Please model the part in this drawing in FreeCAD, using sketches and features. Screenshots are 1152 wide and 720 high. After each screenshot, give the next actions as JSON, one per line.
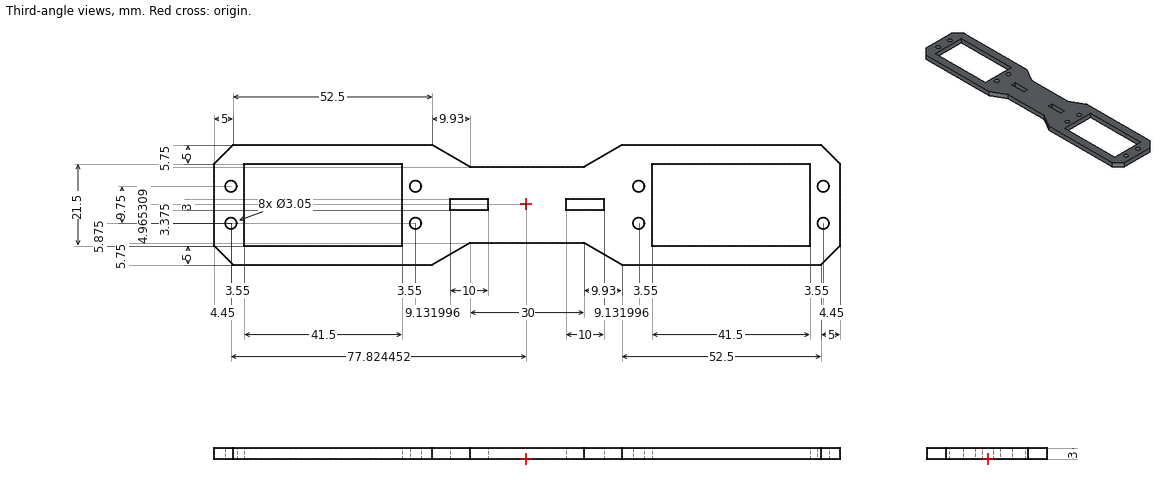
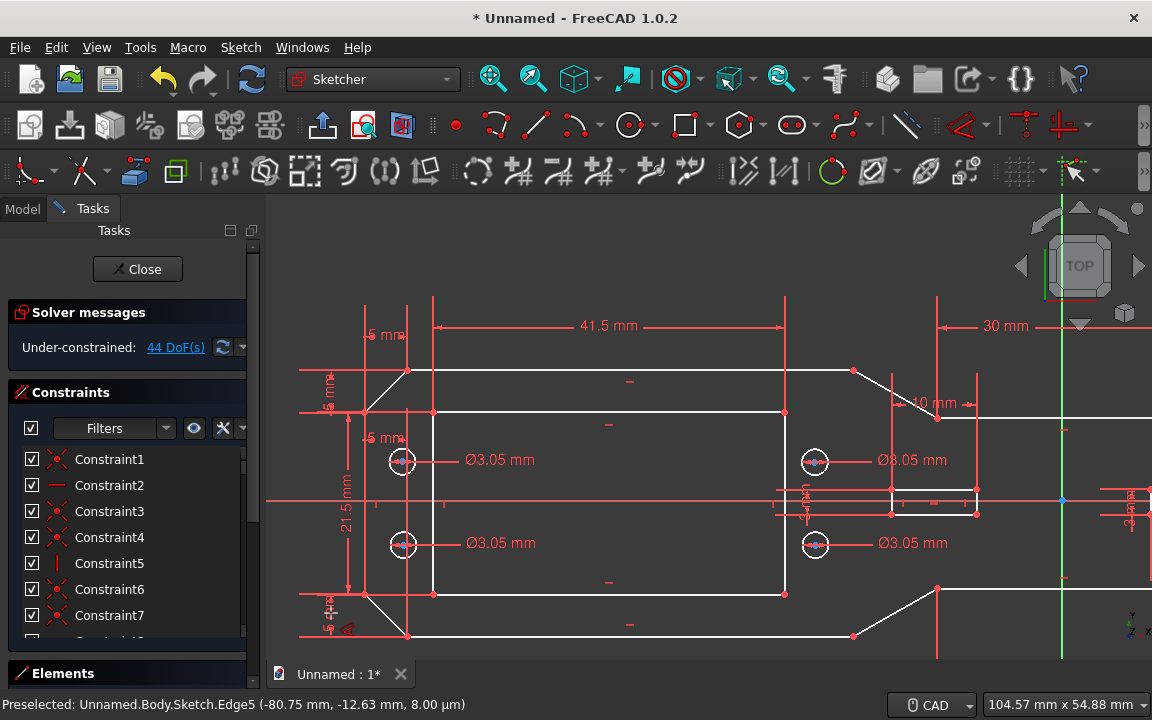
{"action": "scroll", "coordinate": [394, 383], "scroll_direction": "down", "scroll_amount": 5}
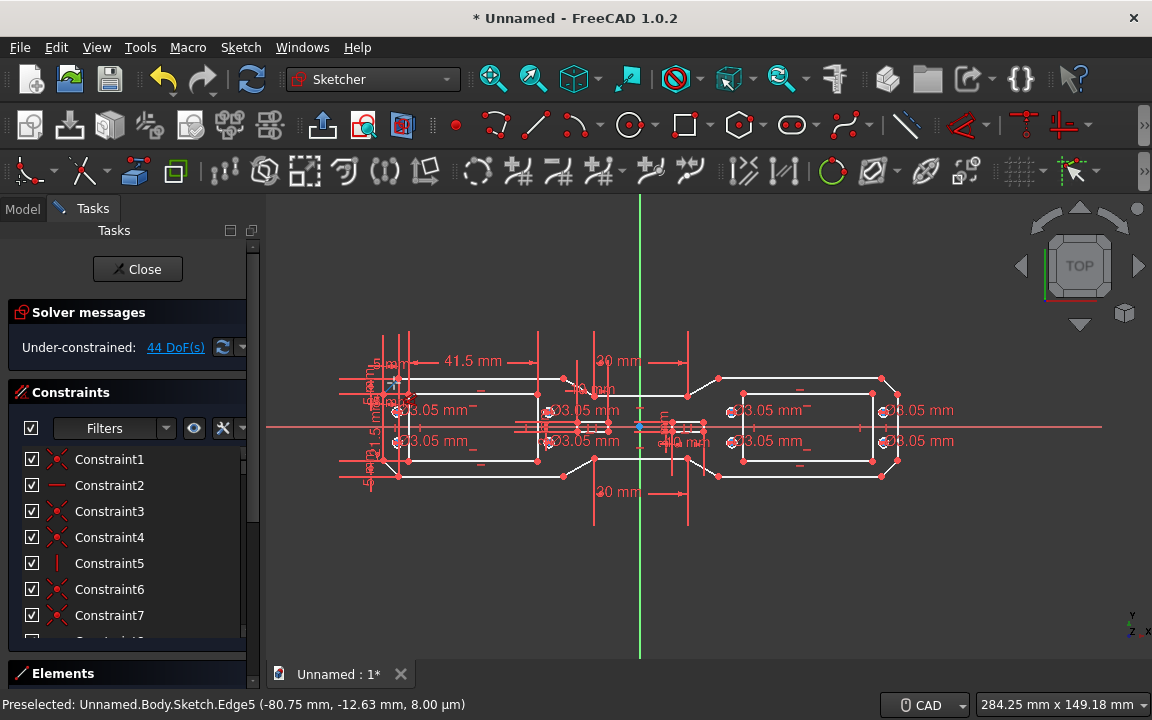
{"action": "scroll", "coordinate": [887, 472], "scroll_direction": "up", "scroll_amount": 5}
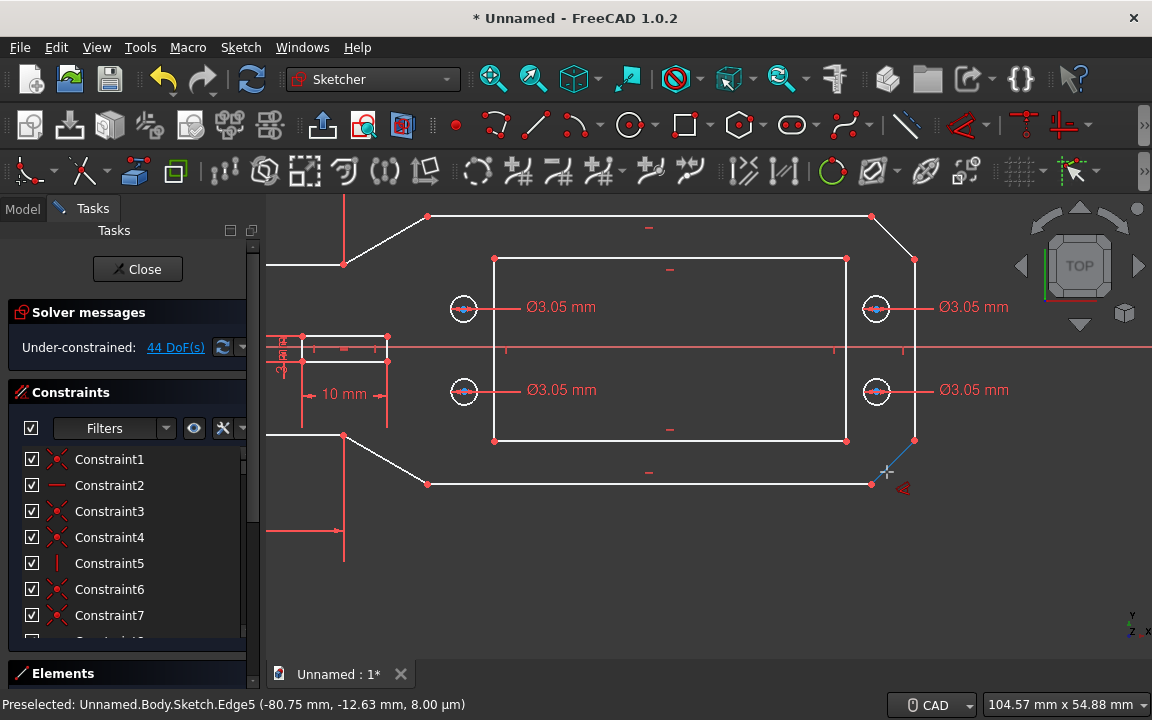
{"action": "left_click", "coordinate": [885, 471]}
{"action": "left_click", "coordinate": [893, 518]}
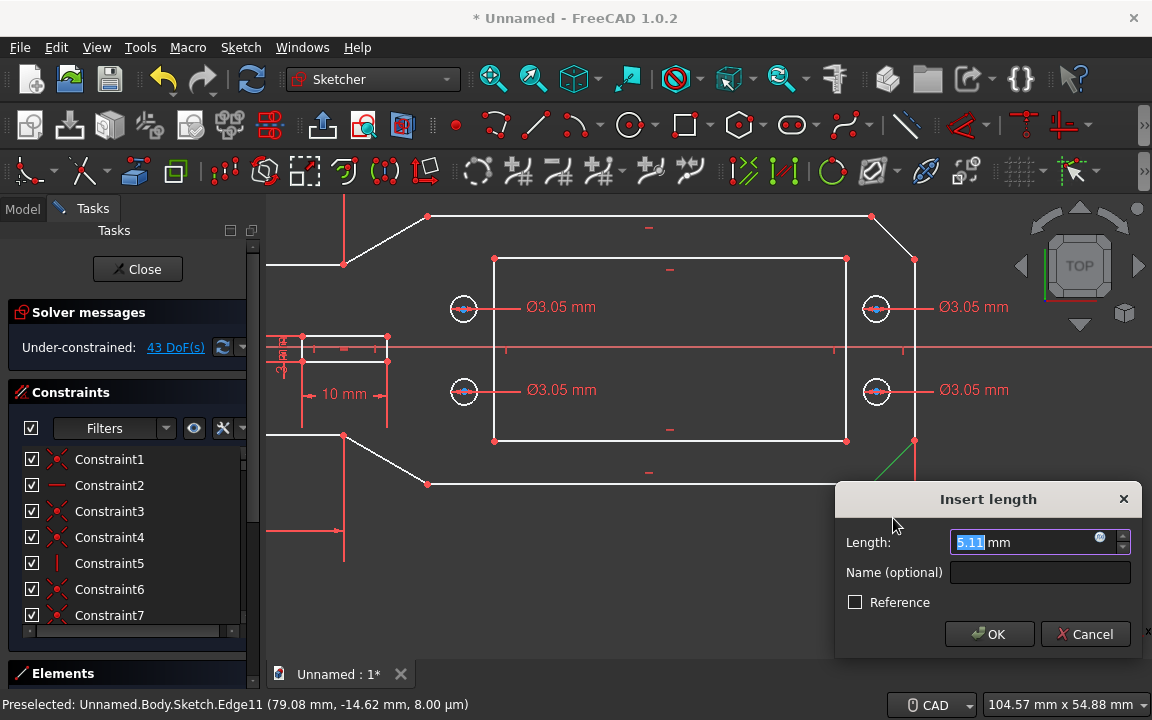
{"action": "type", "text": "5"}
{"action": "key", "text": "Return"}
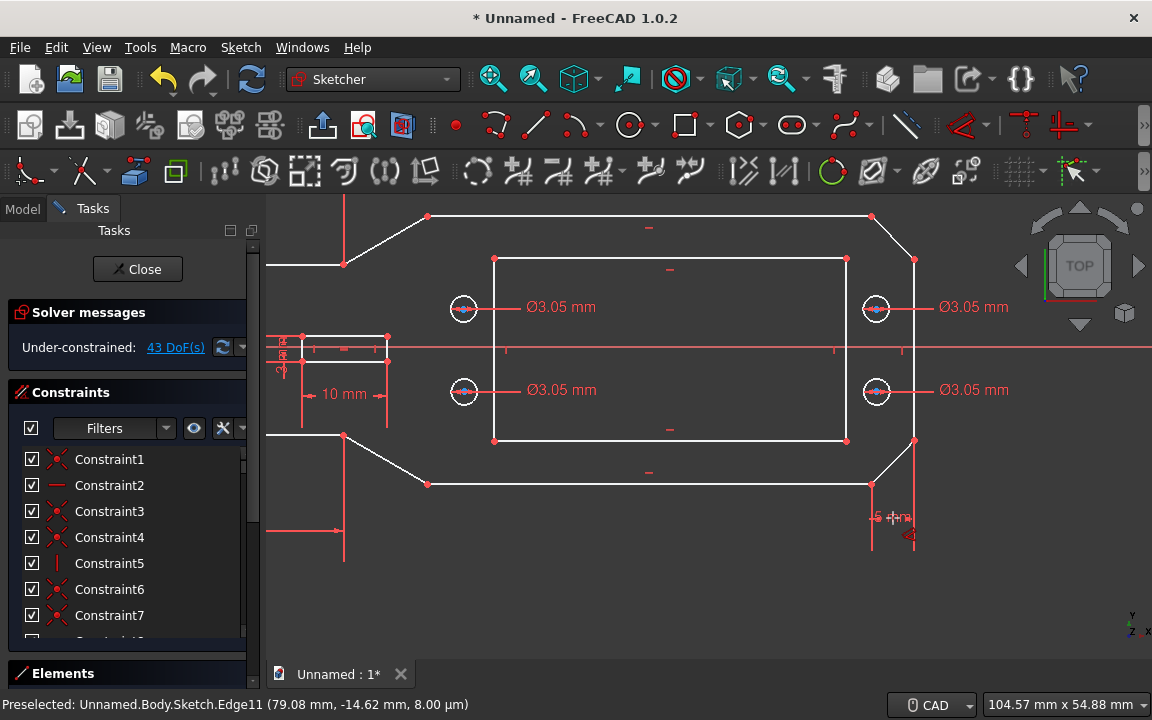
{"action": "left_click", "coordinate": [884, 471]}
{"action": "left_click", "coordinate": [948, 463]}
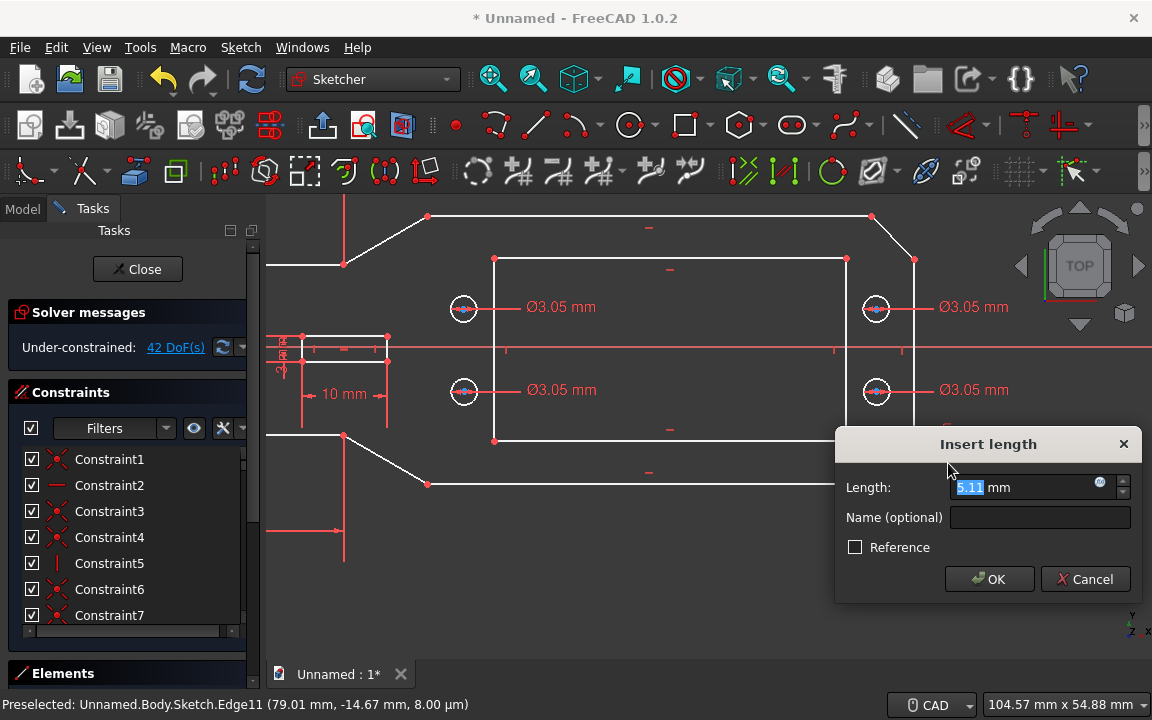
{"action": "type", "text": "5"}
{"action": "key", "text": "Return"}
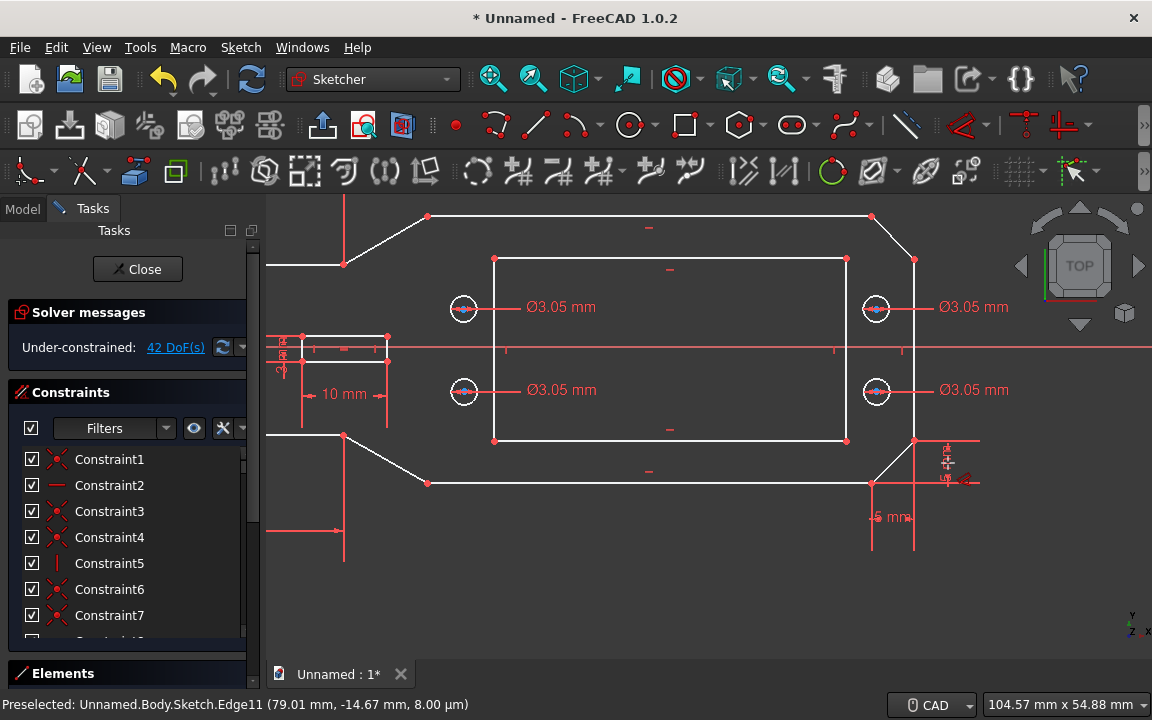
{"action": "left_click", "coordinate": [901, 247]}
{"action": "left_click", "coordinate": [893, 366]}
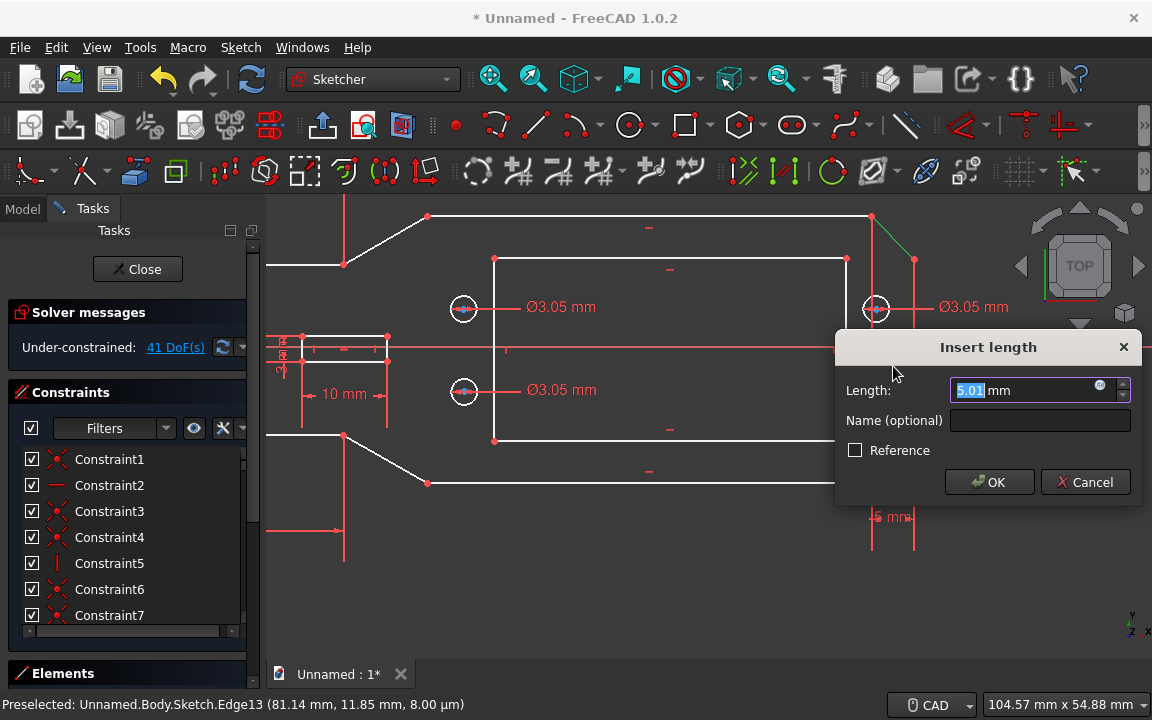
{"action": "type", "text": "5"}
{"action": "key", "text": "Return"}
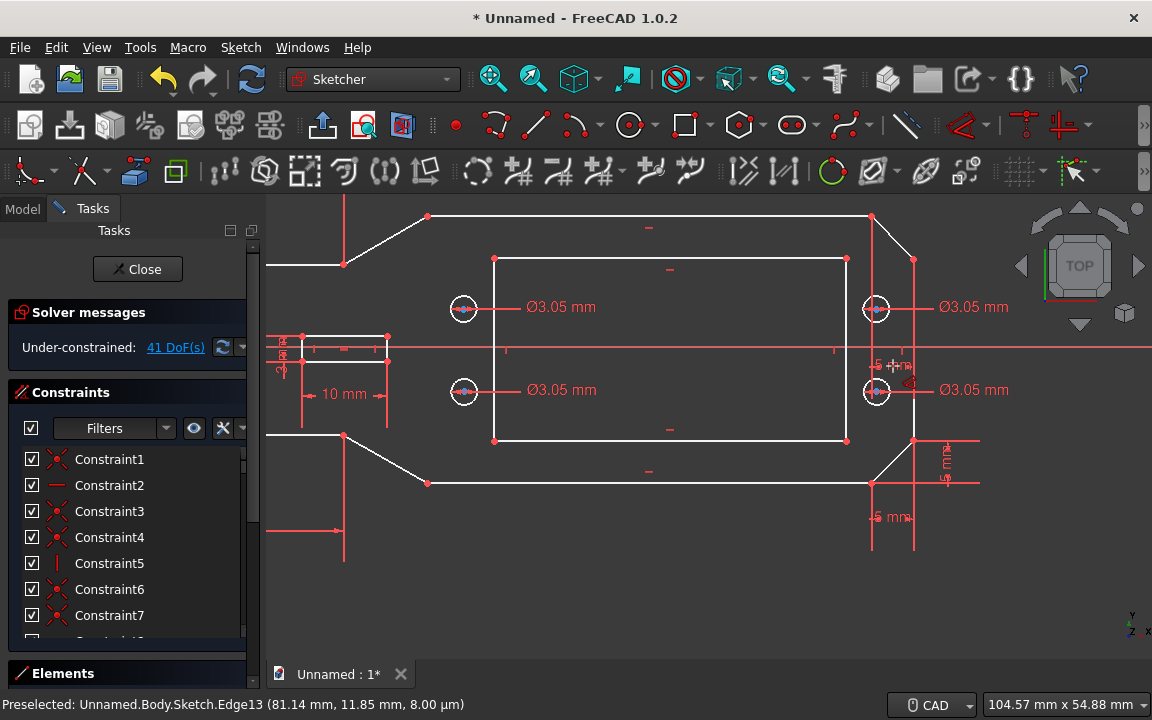
{"action": "left_click", "coordinate": [901, 247]}
{"action": "left_click", "coordinate": [948, 241]}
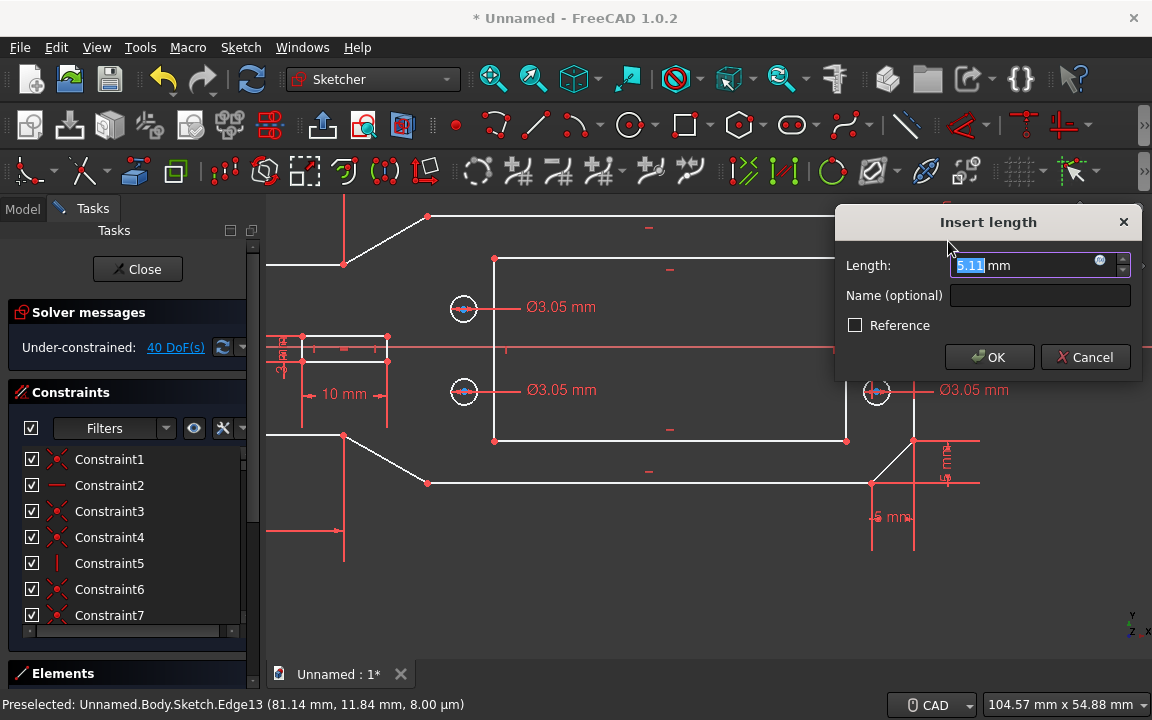
{"action": "type", "text": "5"}
{"action": "key", "text": "Return"}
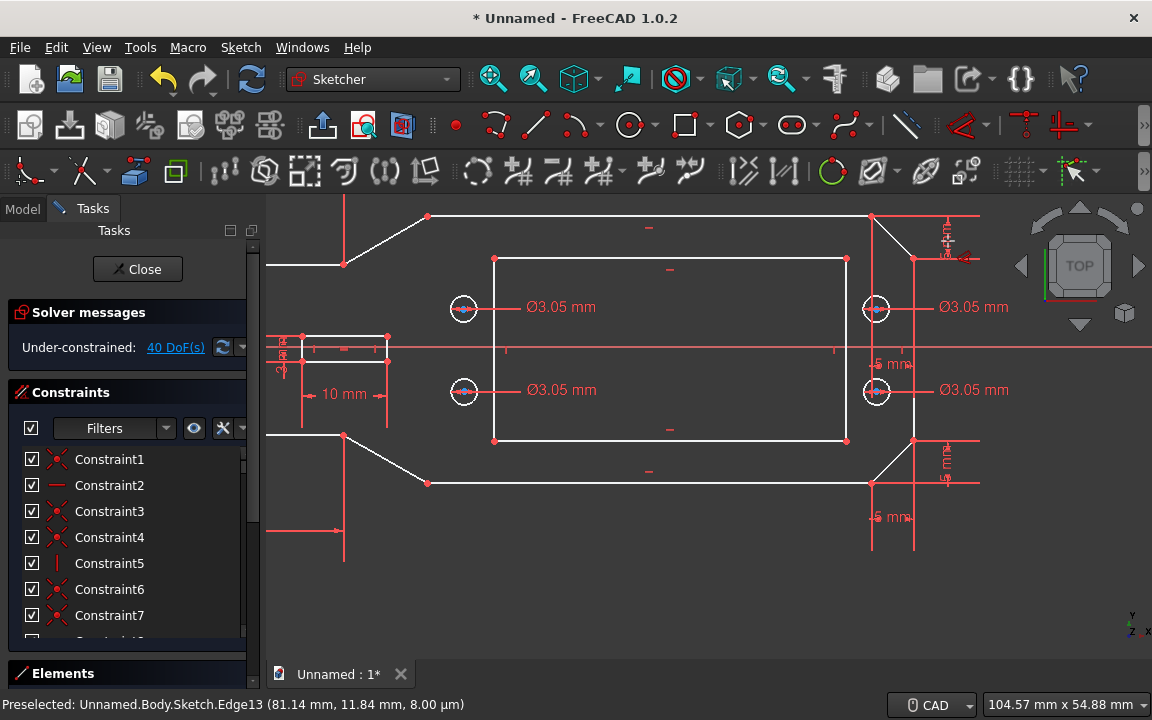
{"action": "scroll", "coordinate": [888, 472], "scroll_direction": "down", "scroll_amount": 5}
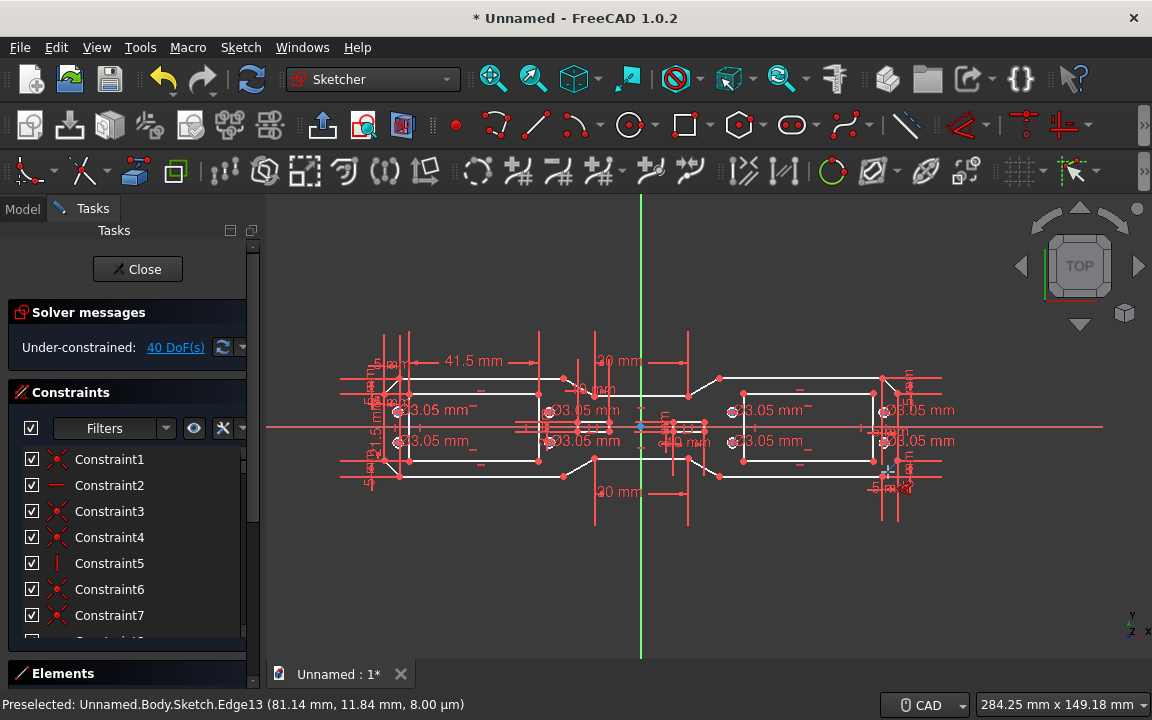
{"action": "left_click", "coordinate": [515, 379]}
{"action": "left_click", "coordinate": [482, 345]}